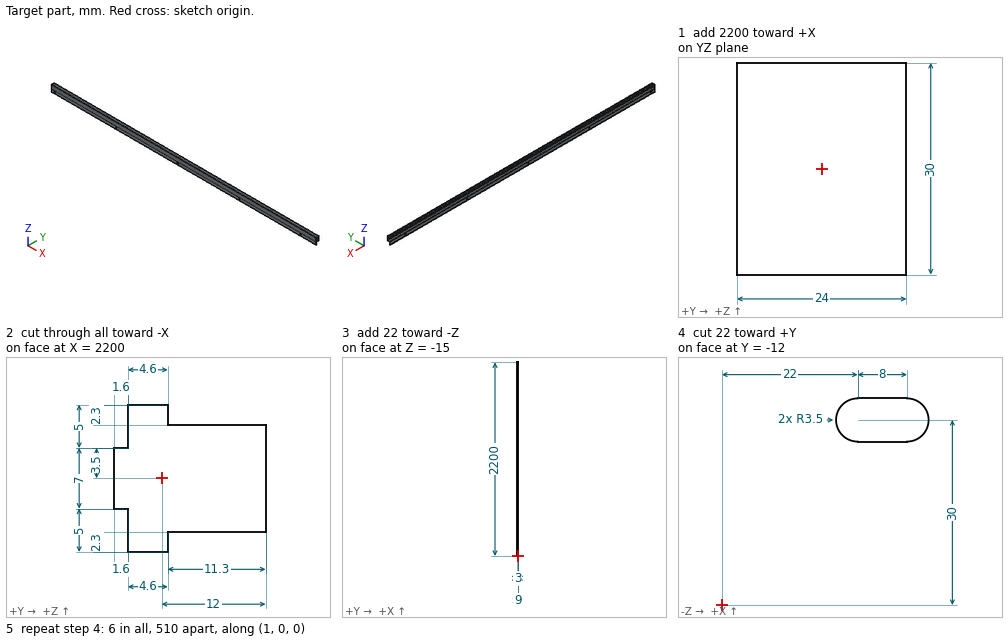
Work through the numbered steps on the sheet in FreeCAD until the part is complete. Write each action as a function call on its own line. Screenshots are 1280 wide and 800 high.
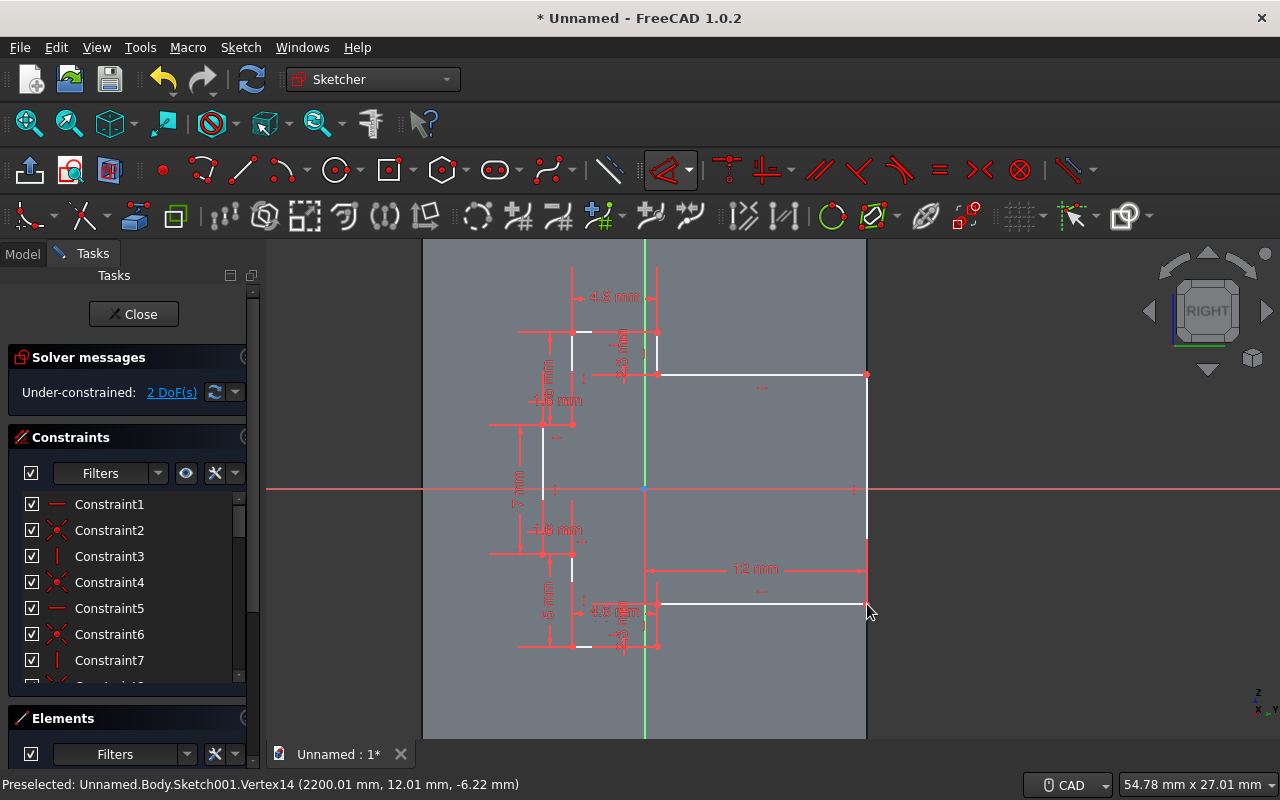
click(720, 604)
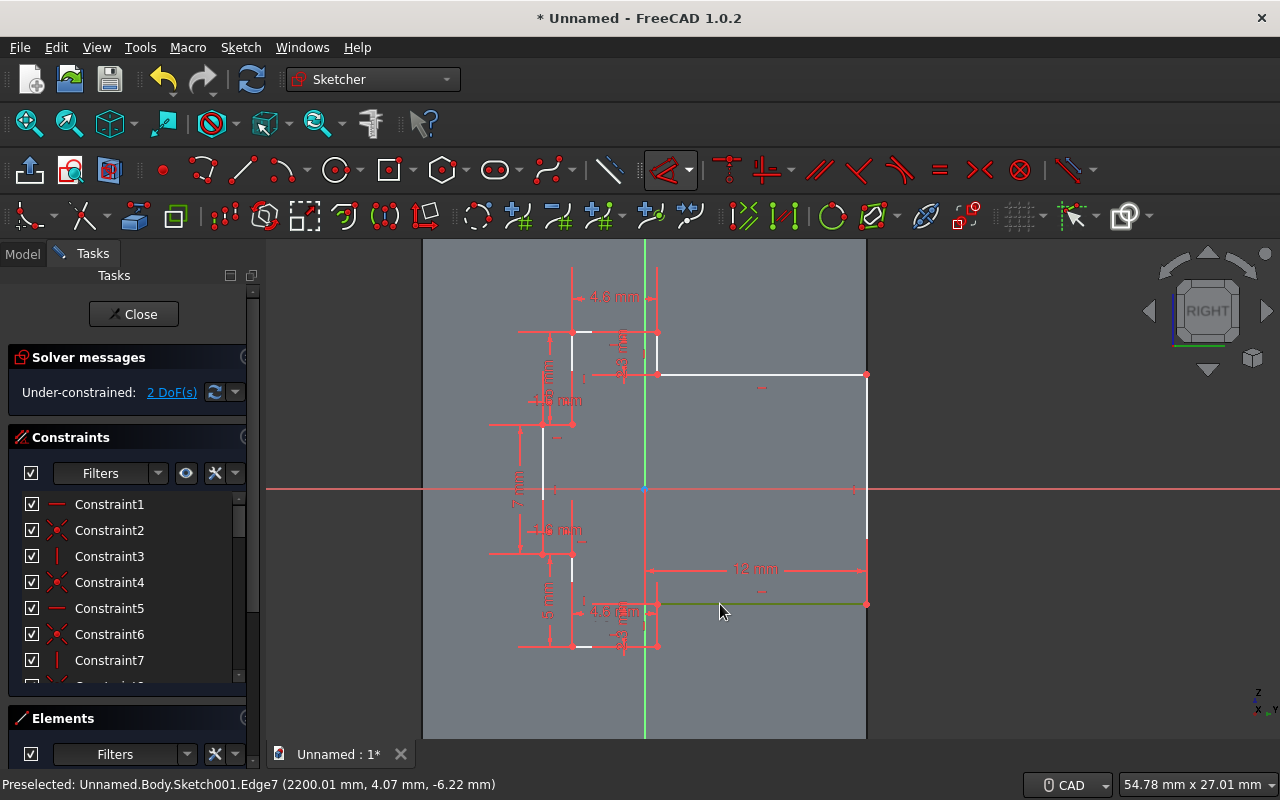
click(692, 170)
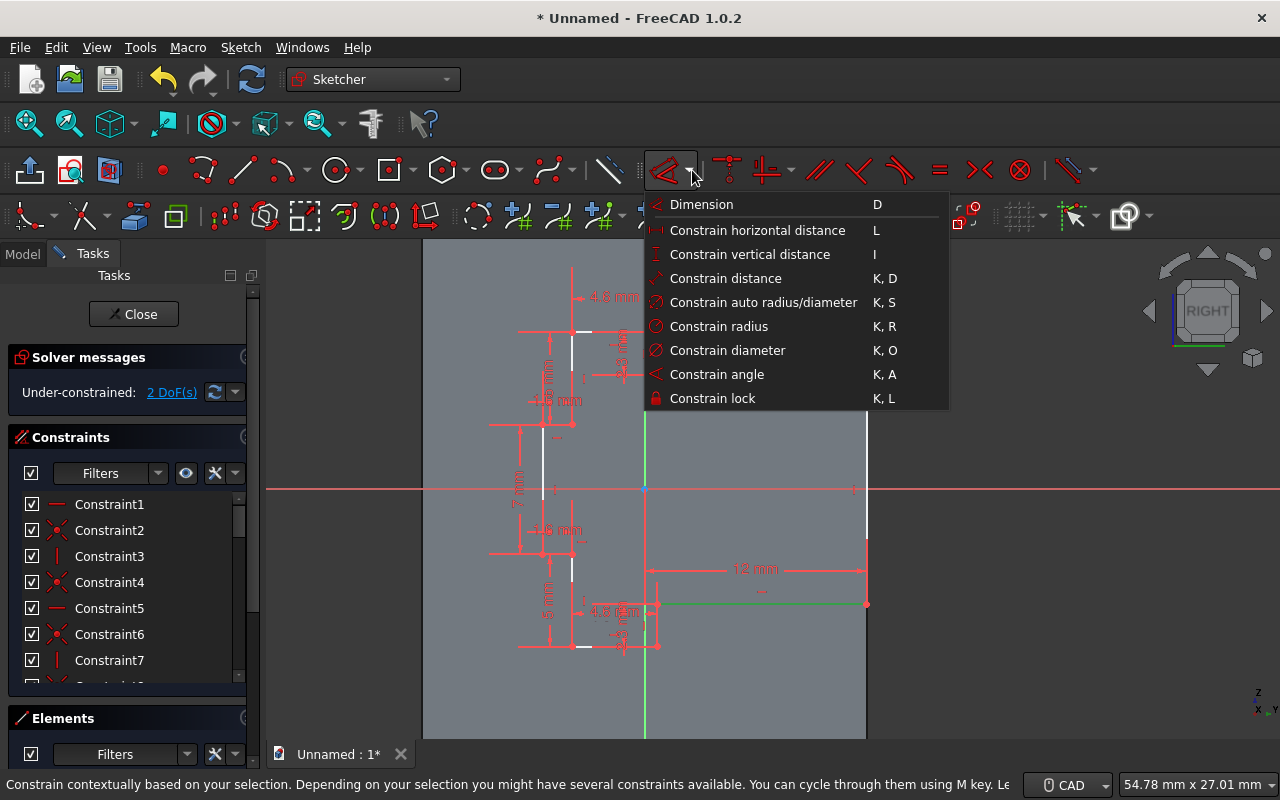
click(797, 230)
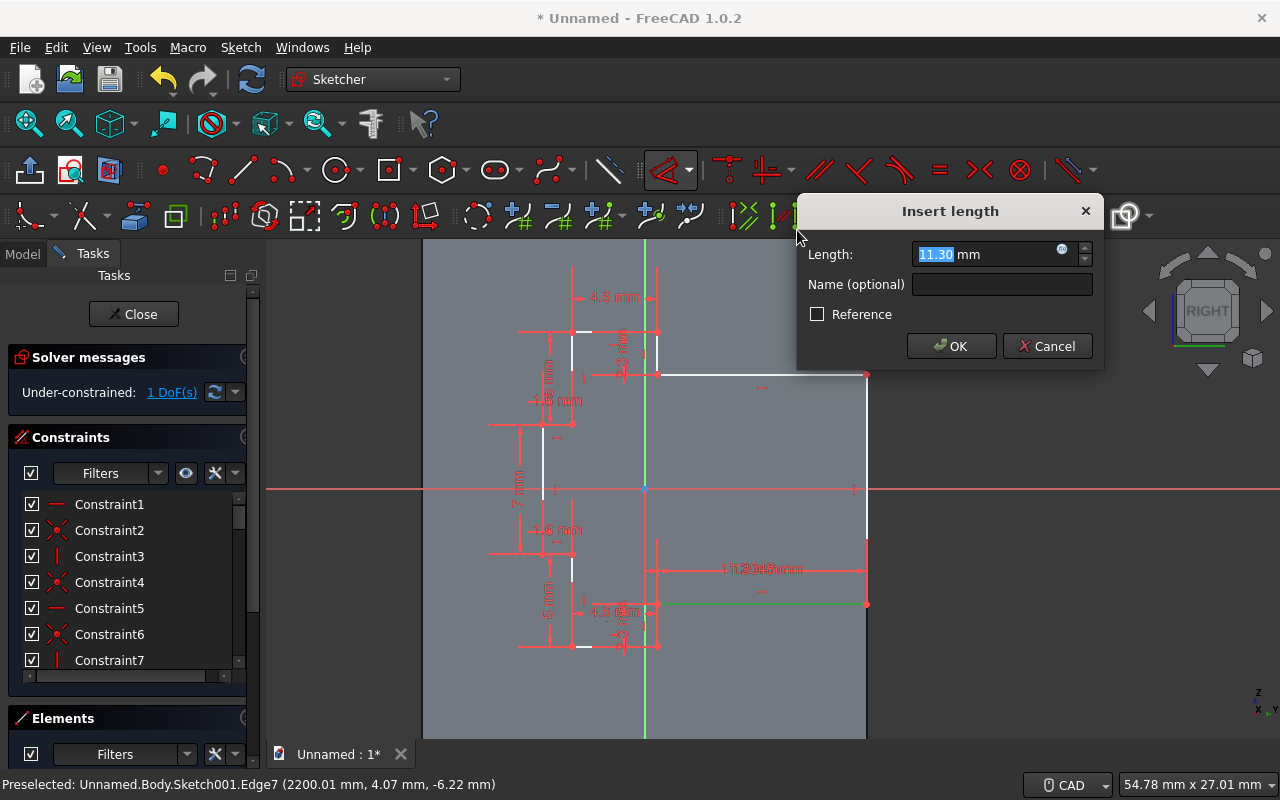
text(11.3)
key(Return)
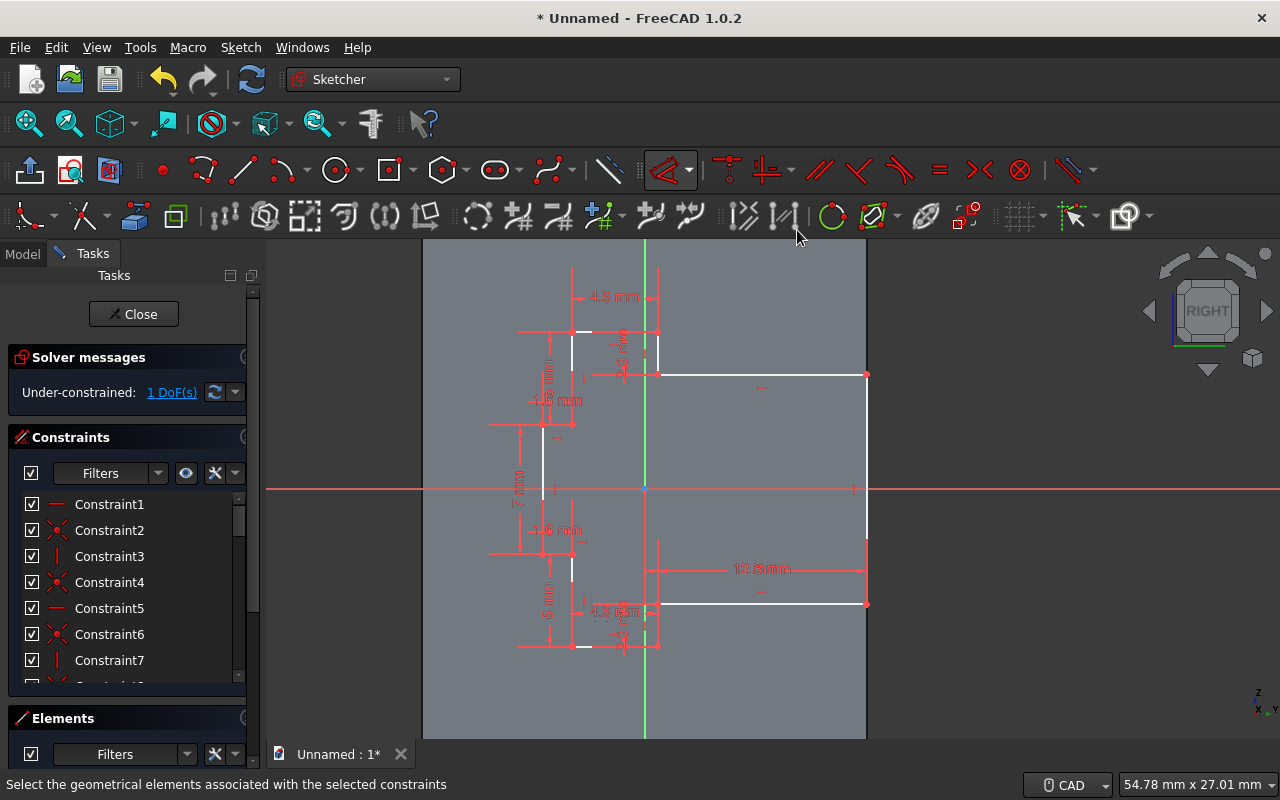
click(572, 425)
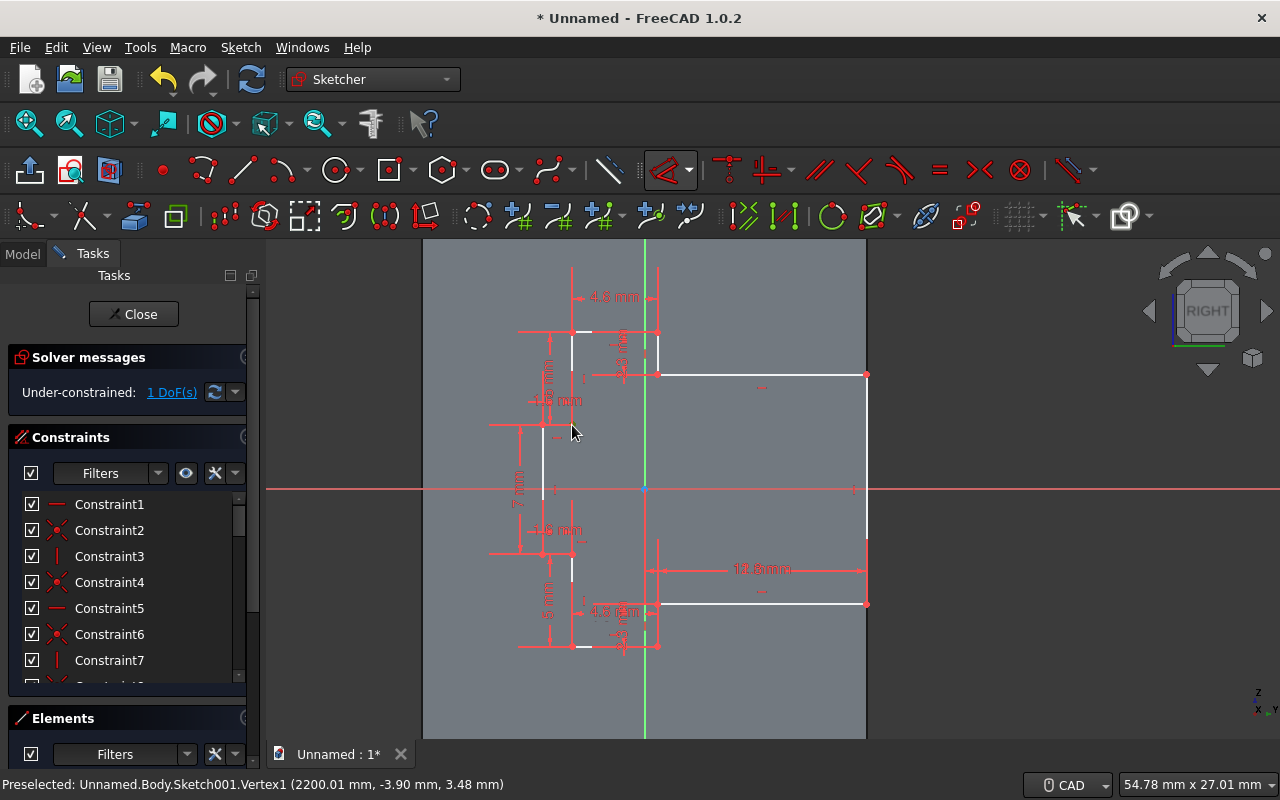
key(i)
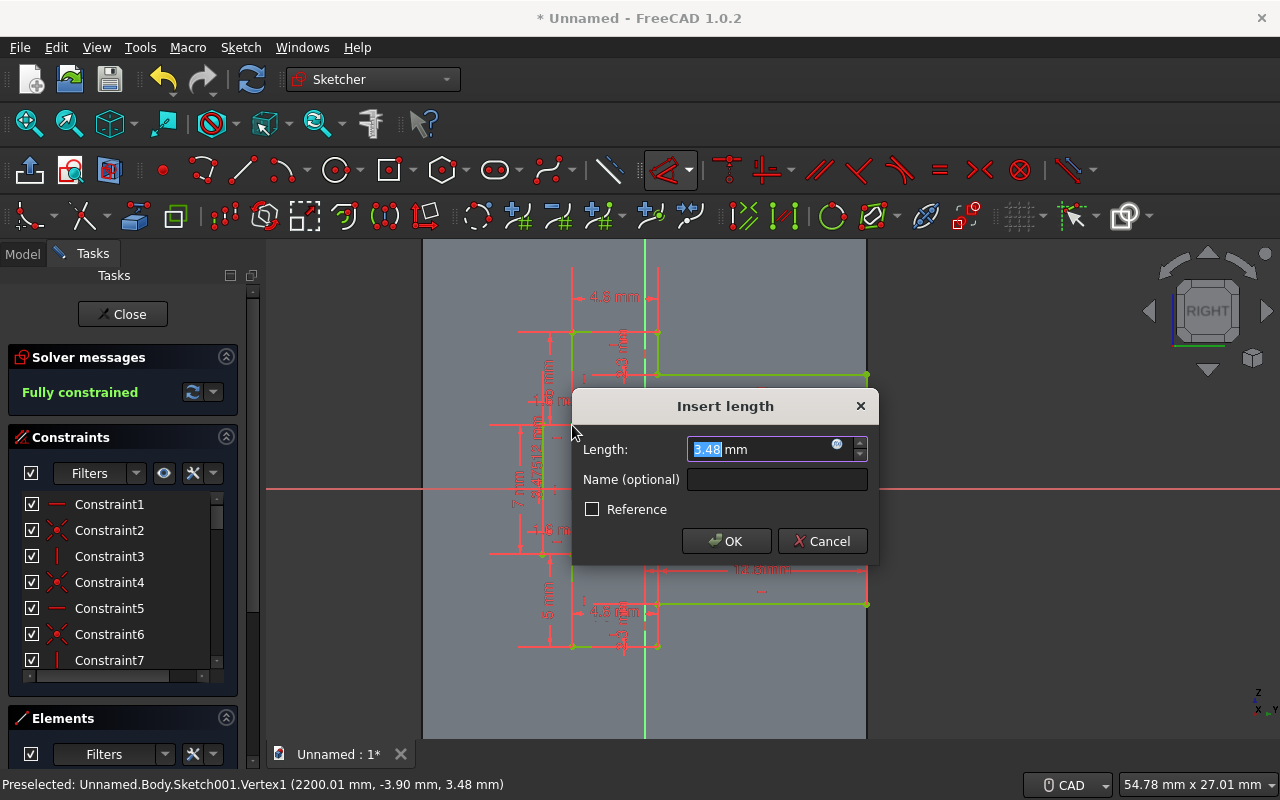
text(3.5)
key(Return)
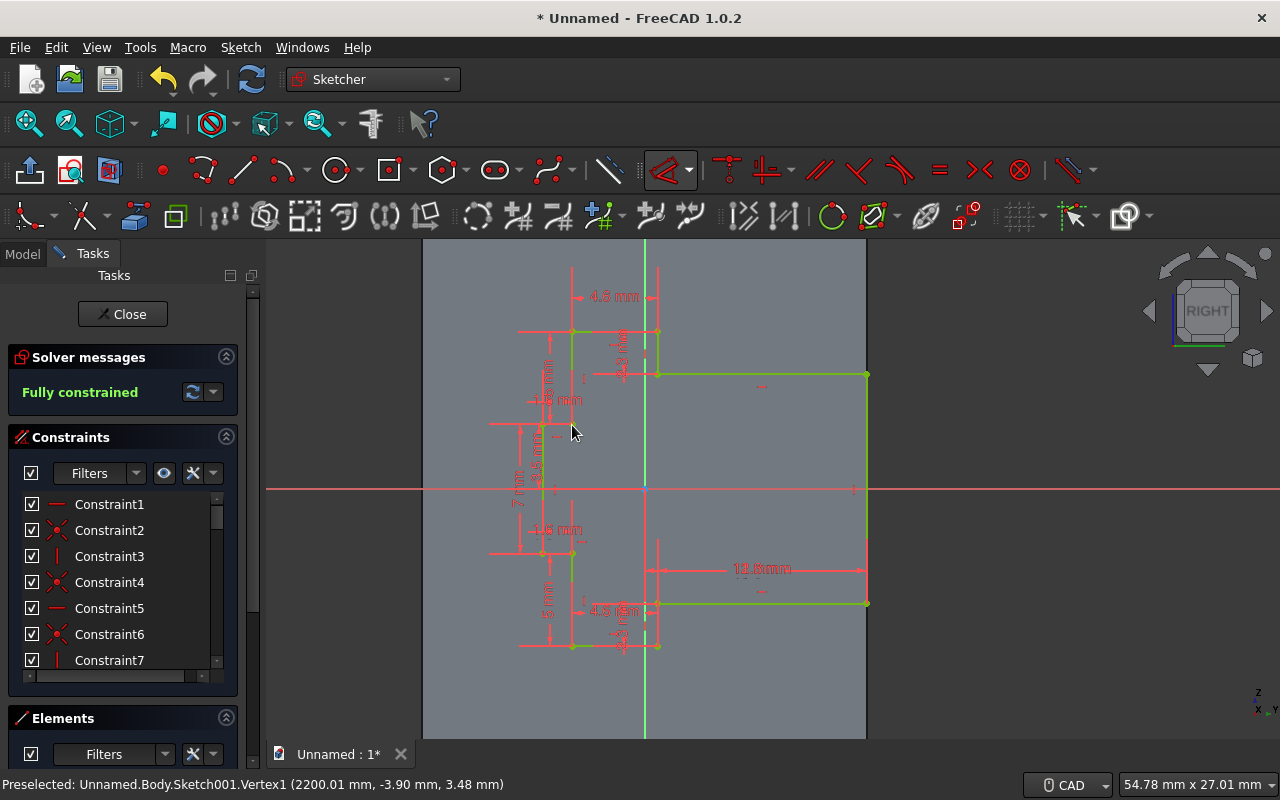
click(123, 314)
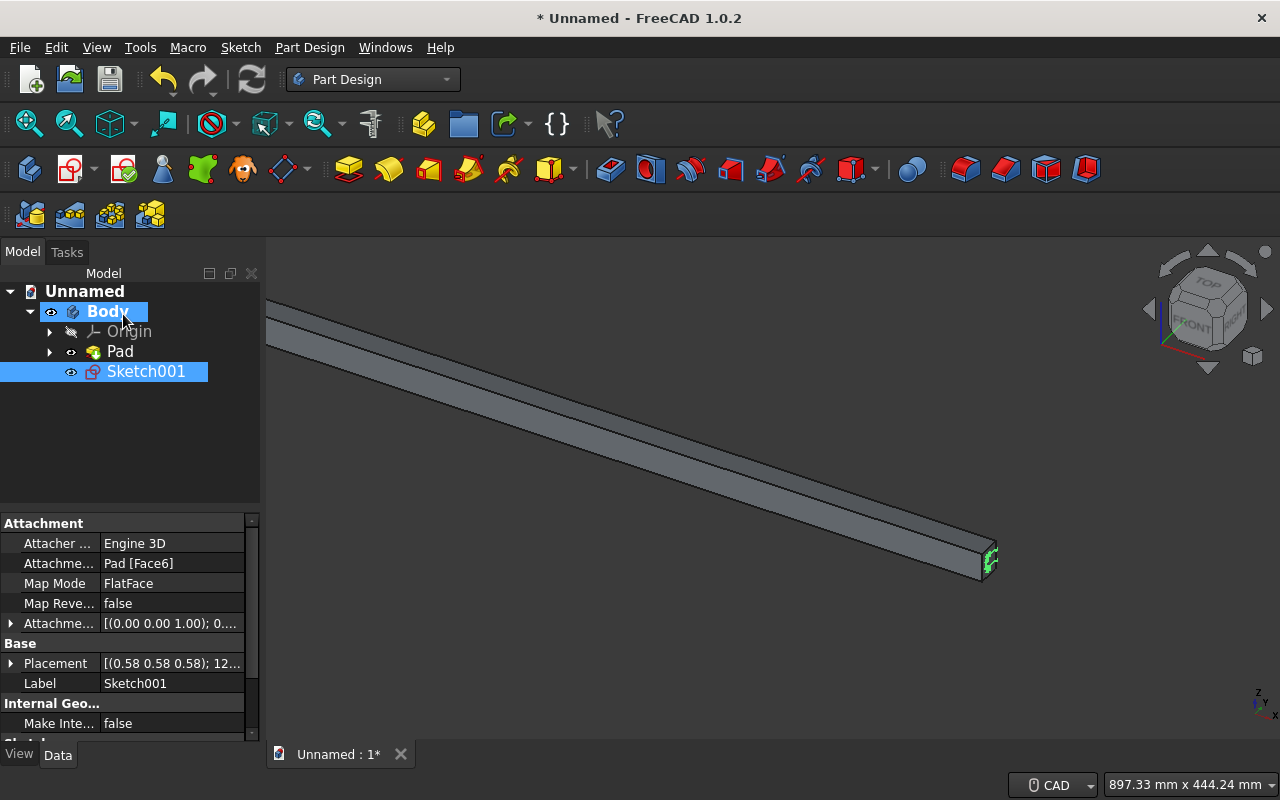
click(612, 170)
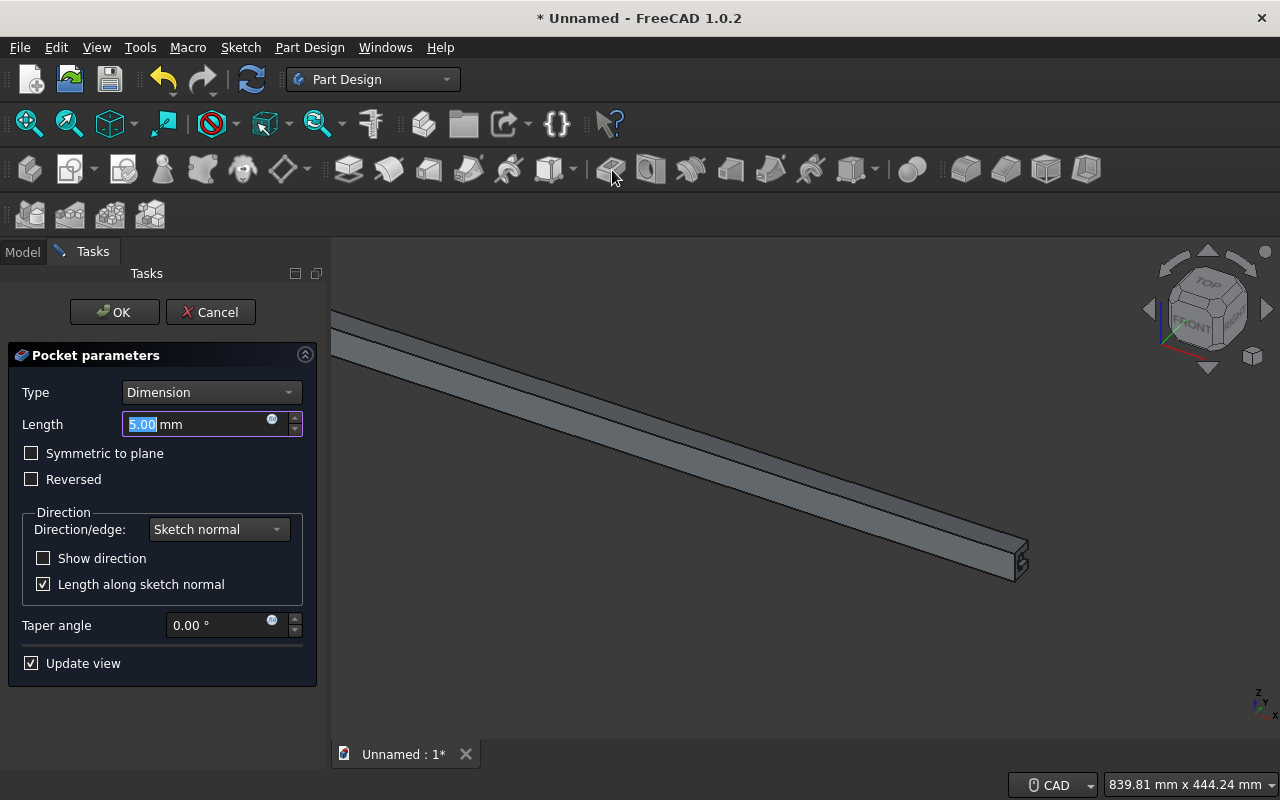
click(212, 392)